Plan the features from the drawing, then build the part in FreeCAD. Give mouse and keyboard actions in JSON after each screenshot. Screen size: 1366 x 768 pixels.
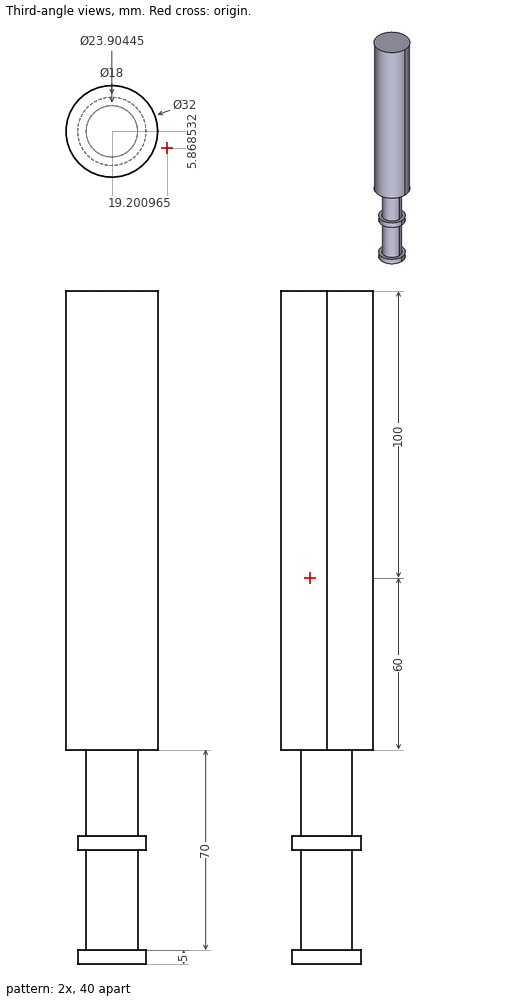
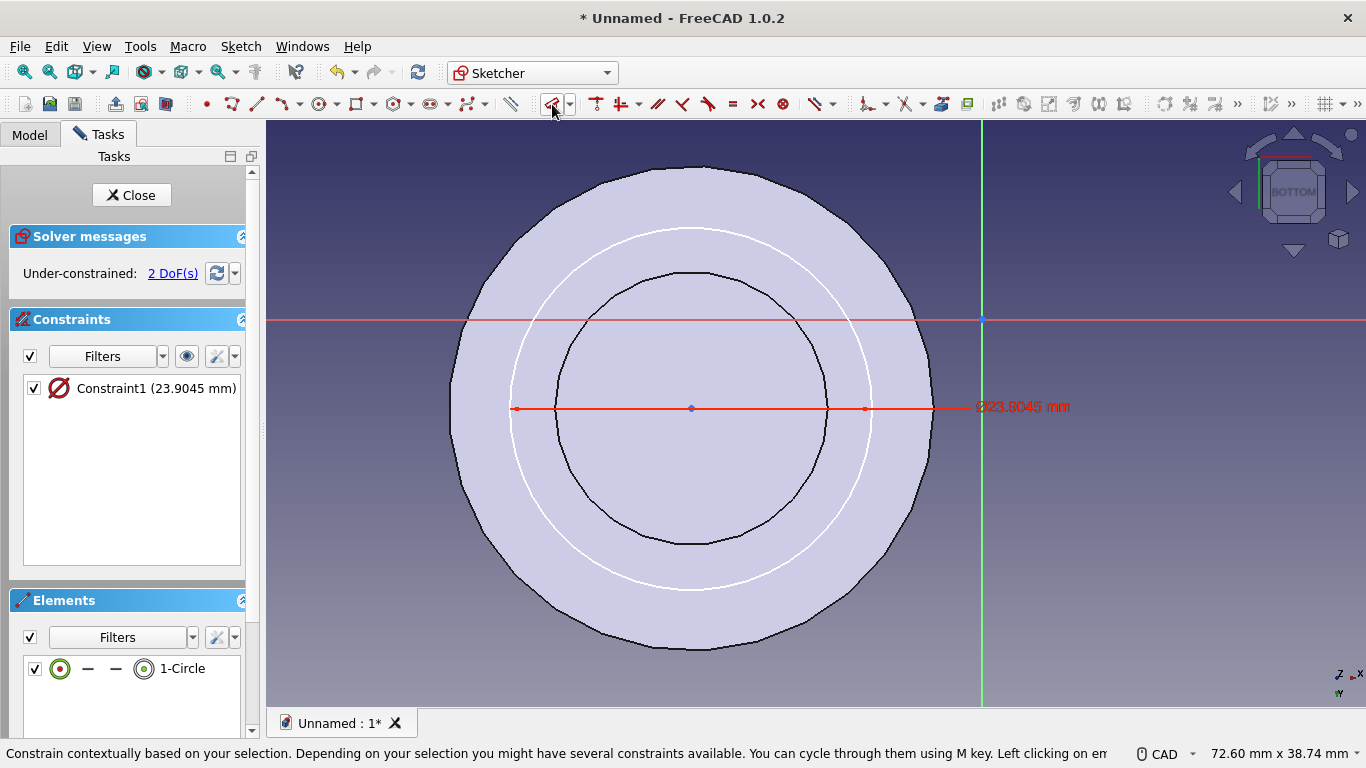
{"action": "left_click", "coordinate": [691, 409]}
{"action": "left_click", "coordinate": [1016, 364]}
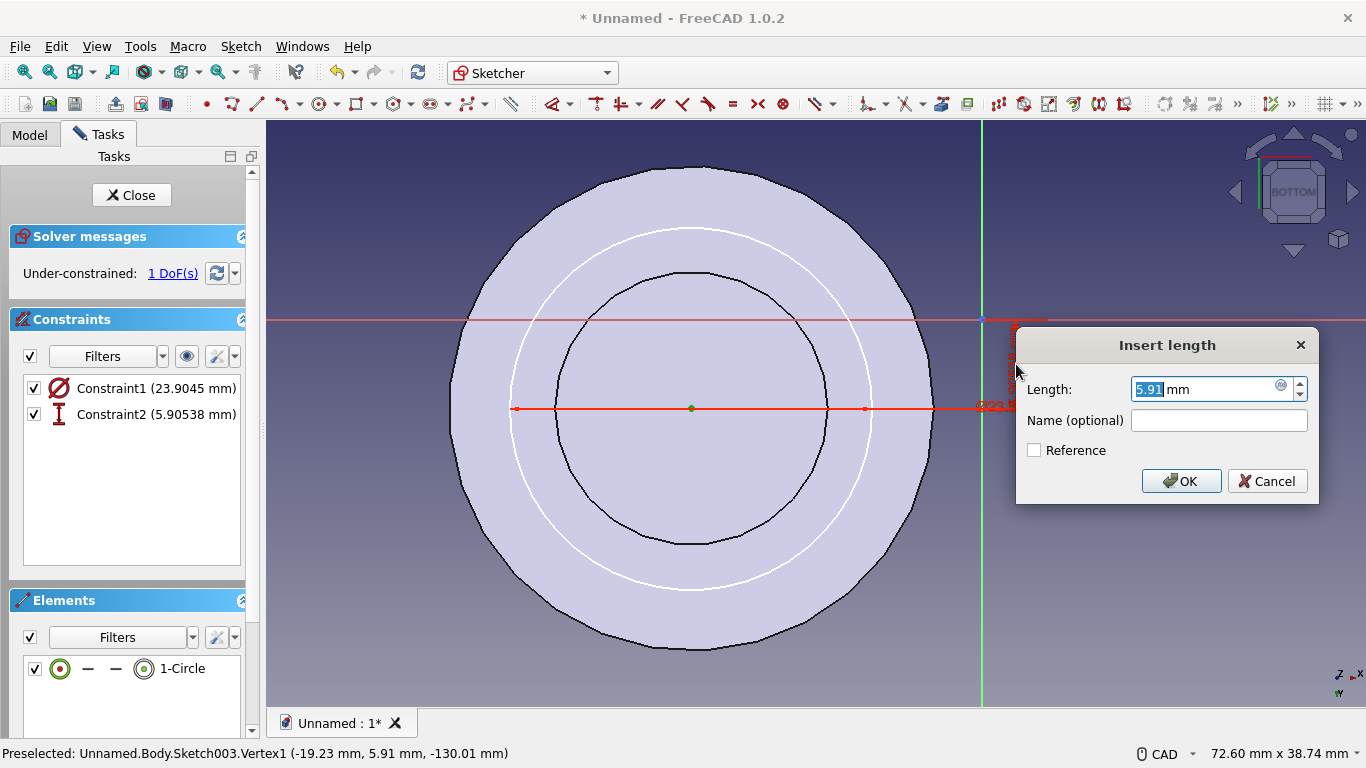
{"action": "type", "text": "5.868532"}
{"action": "key", "text": "Return"}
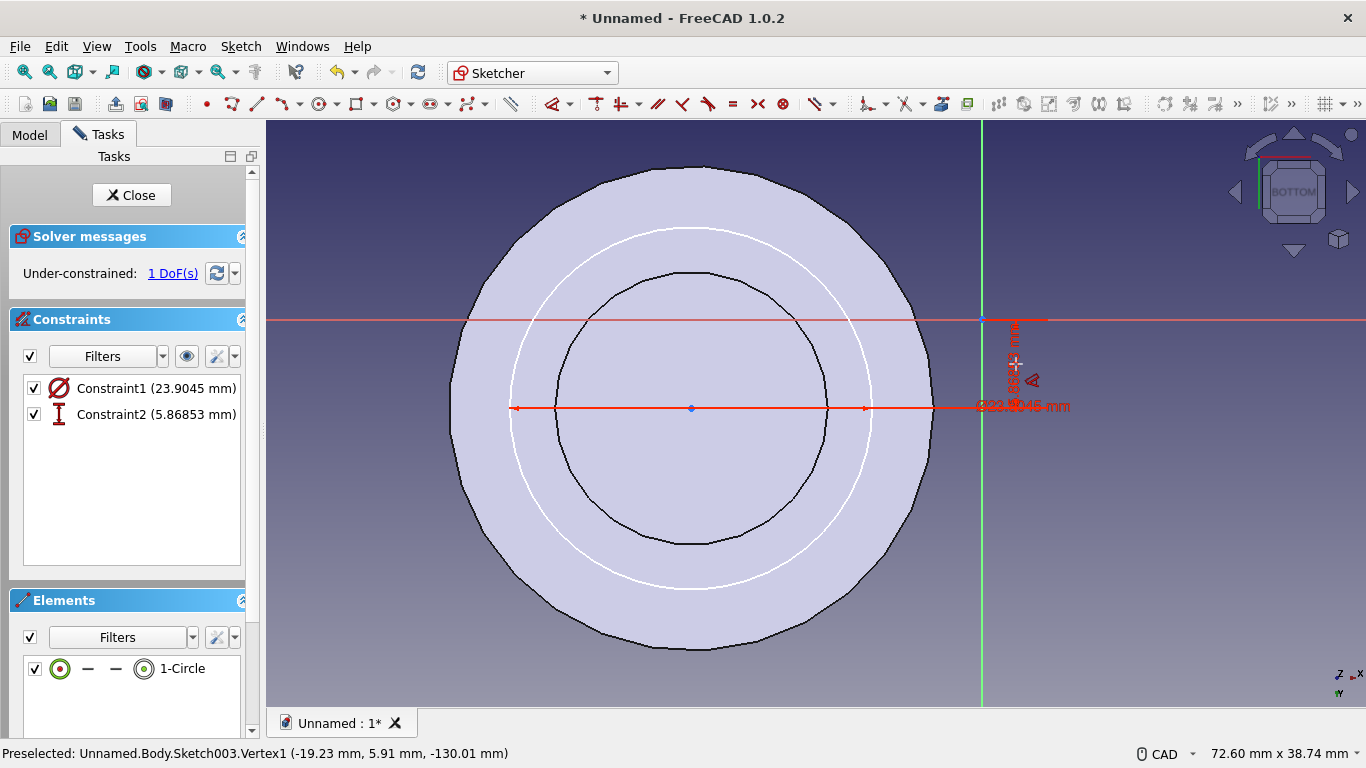
{"action": "left_click", "coordinate": [691, 408]}
{"action": "left_click", "coordinate": [770, 286]}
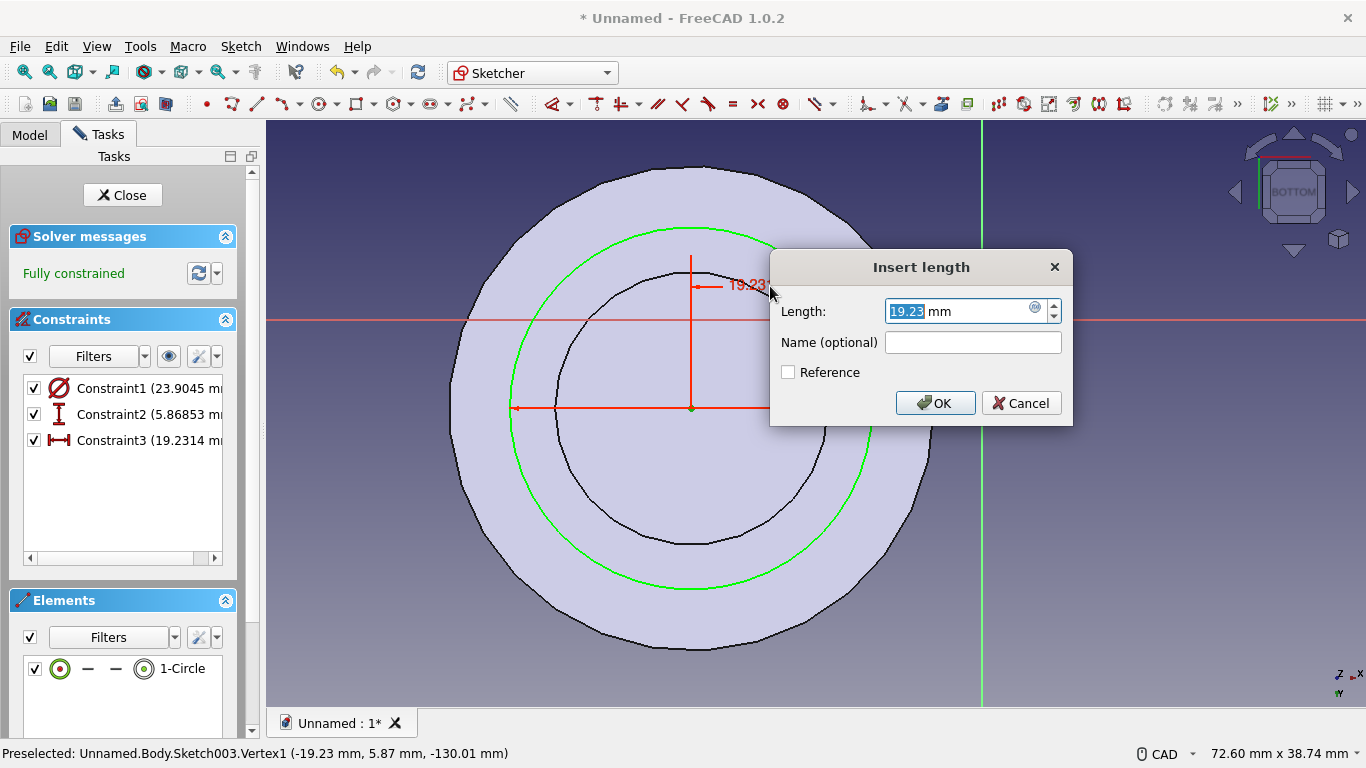
{"action": "type", "text": "19.200965"}
{"action": "key", "text": "Return"}
{"action": "key", "text": "Escape"}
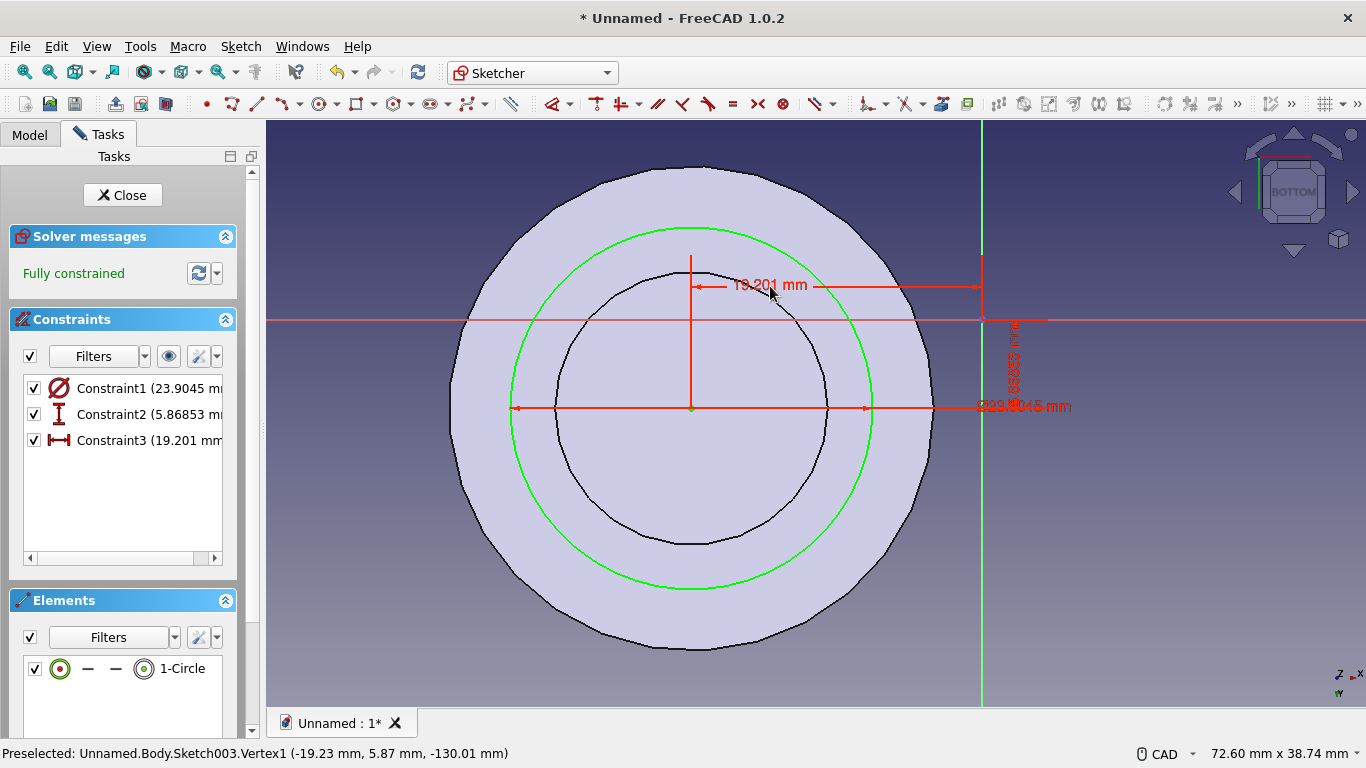
{"action": "left_click", "coordinate": [123, 195]}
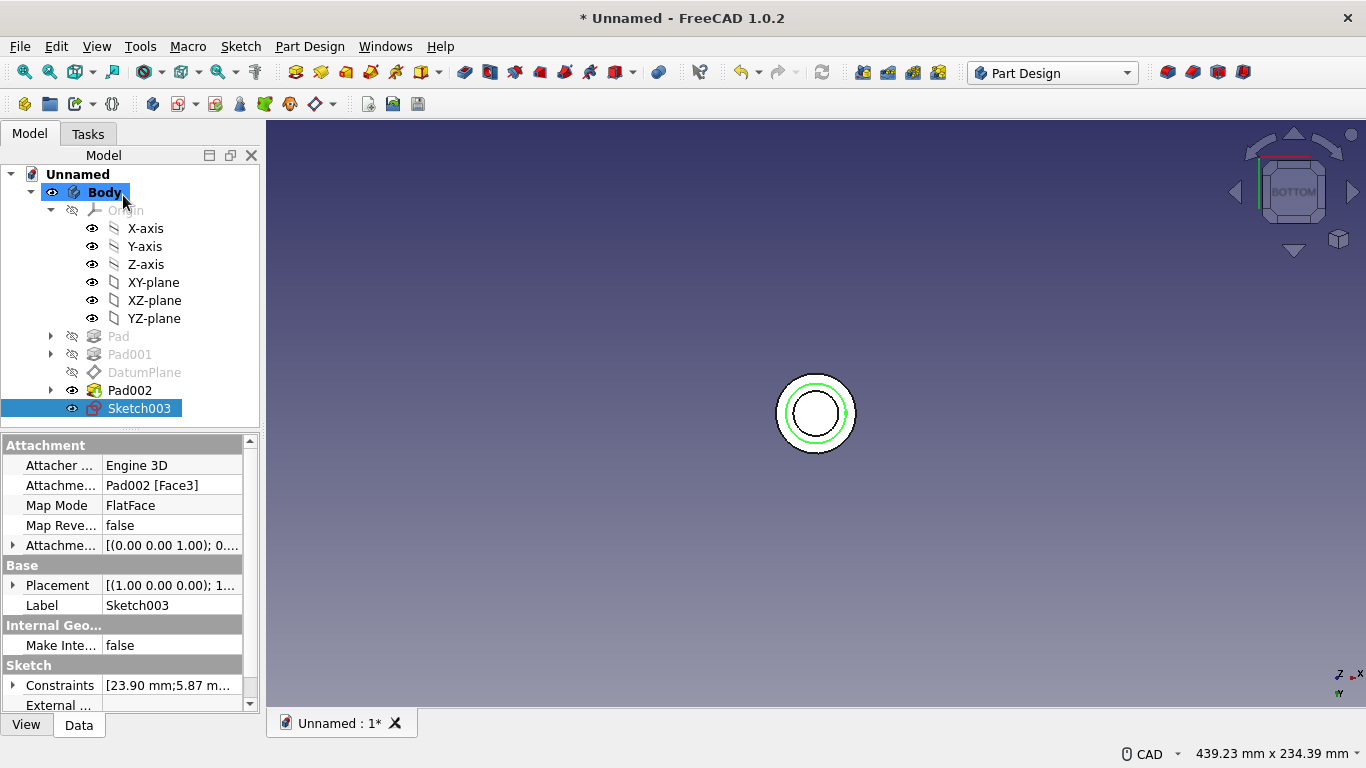
{"action": "left_click", "coordinate": [296, 72]}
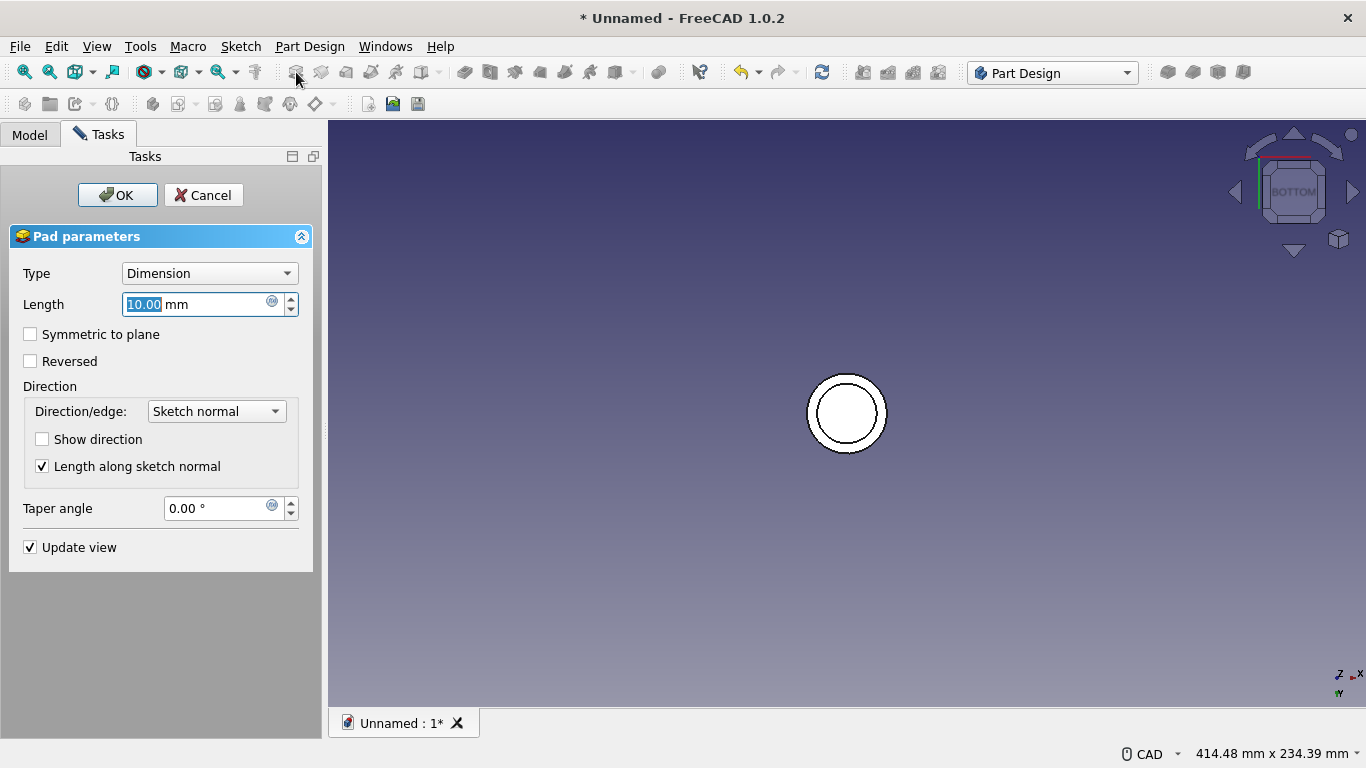
{"action": "type", "text": "5"}
{"action": "key", "text": "Tab"}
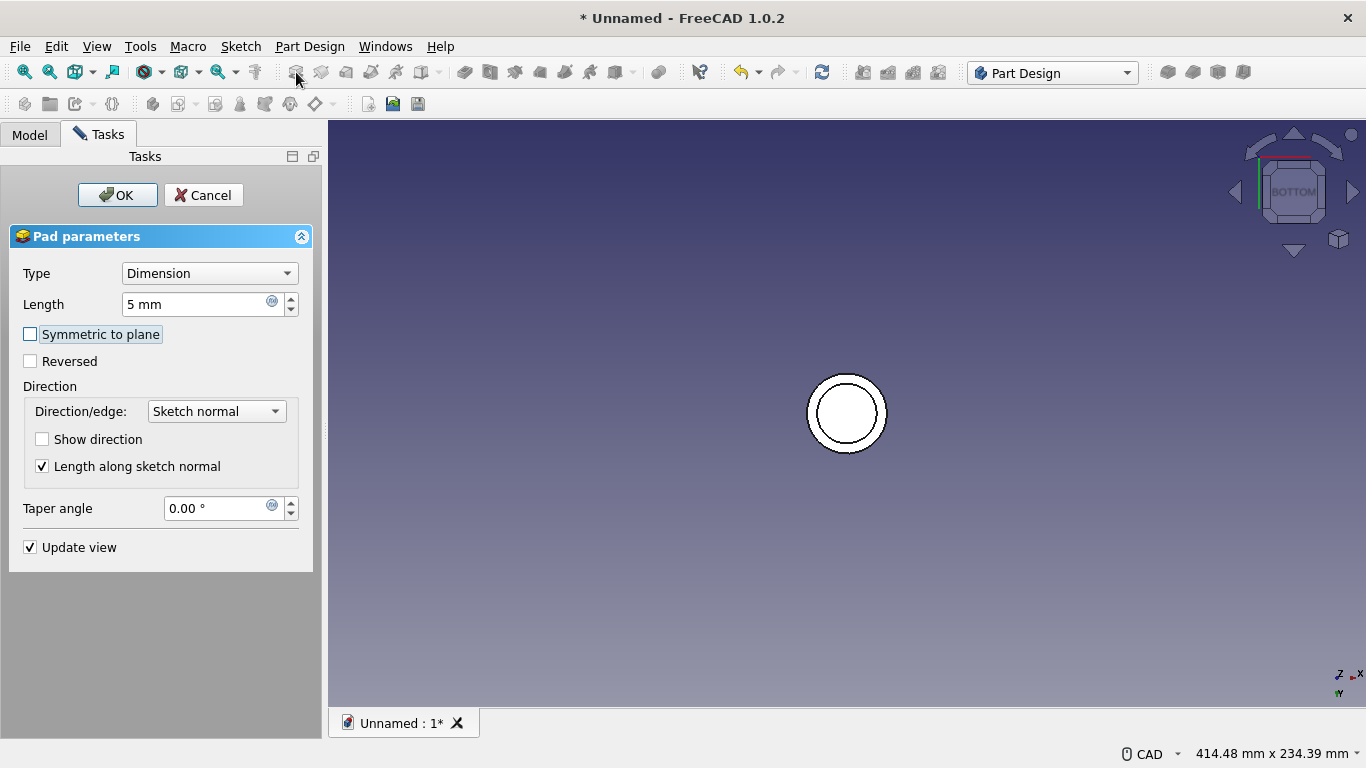
{"action": "left_click", "coordinate": [118, 195]}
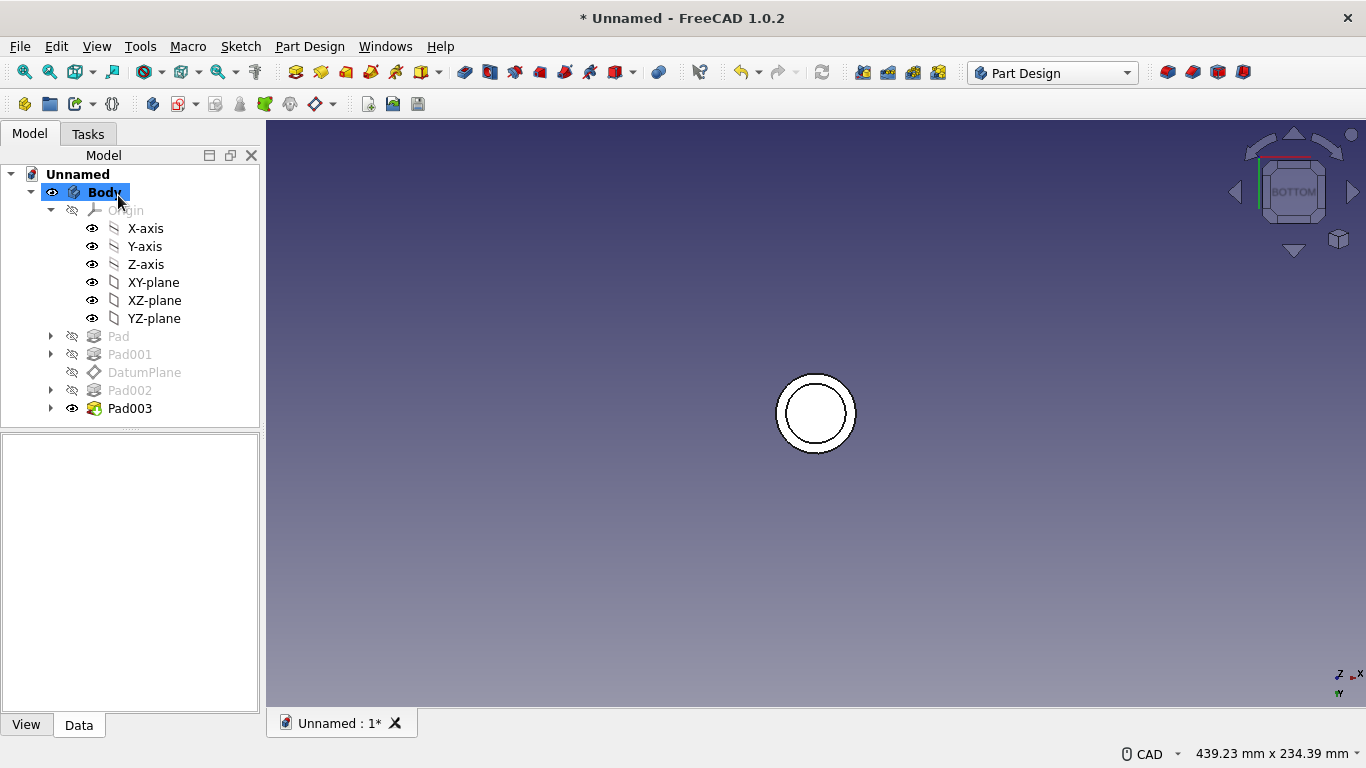
{"action": "left_click", "coordinate": [25, 72]}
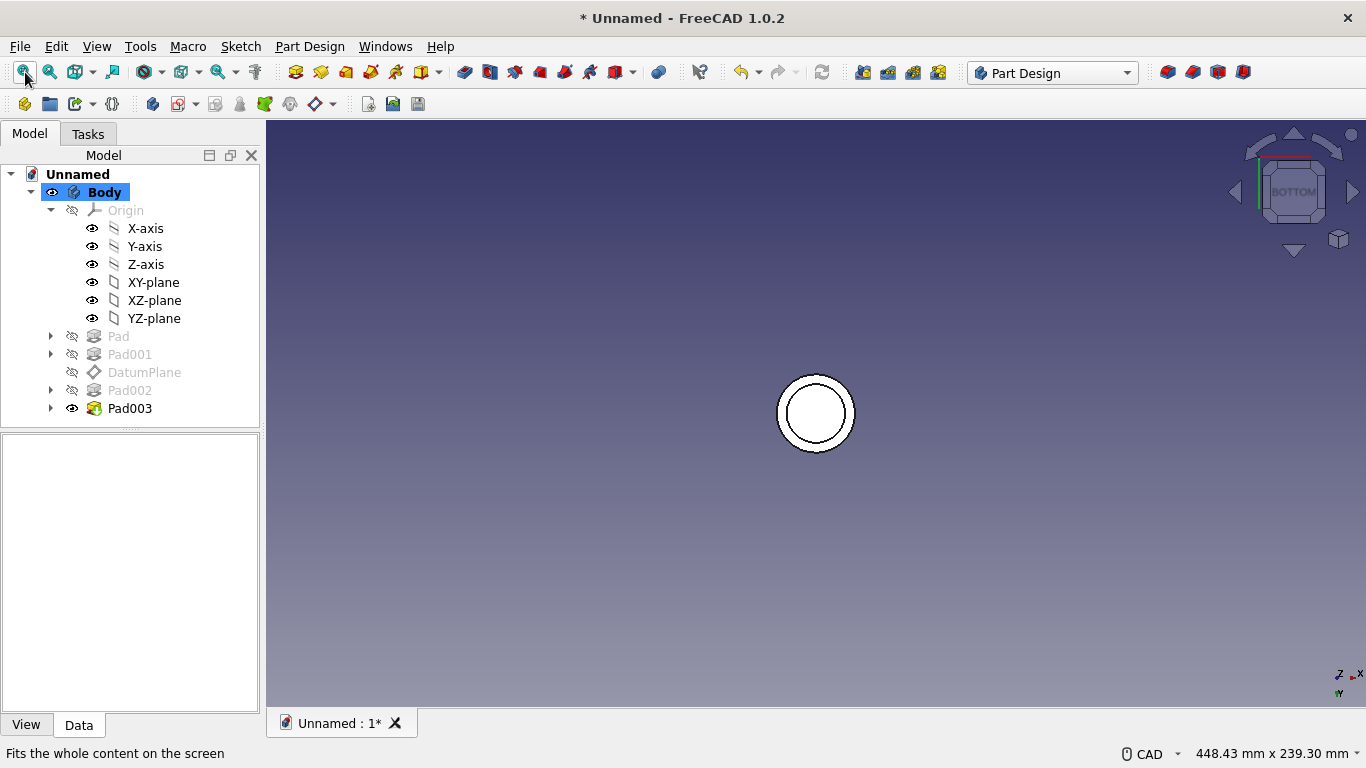
{"action": "left_click", "coordinate": [117, 408]}